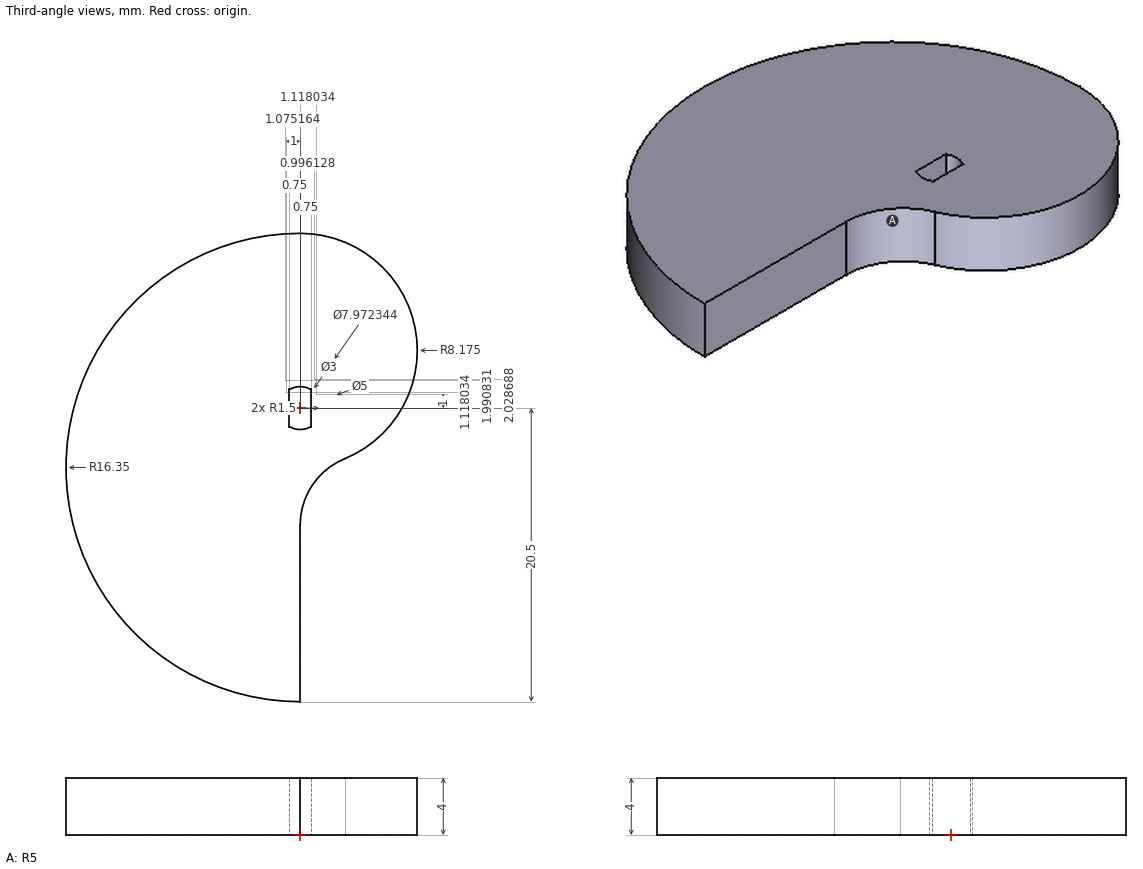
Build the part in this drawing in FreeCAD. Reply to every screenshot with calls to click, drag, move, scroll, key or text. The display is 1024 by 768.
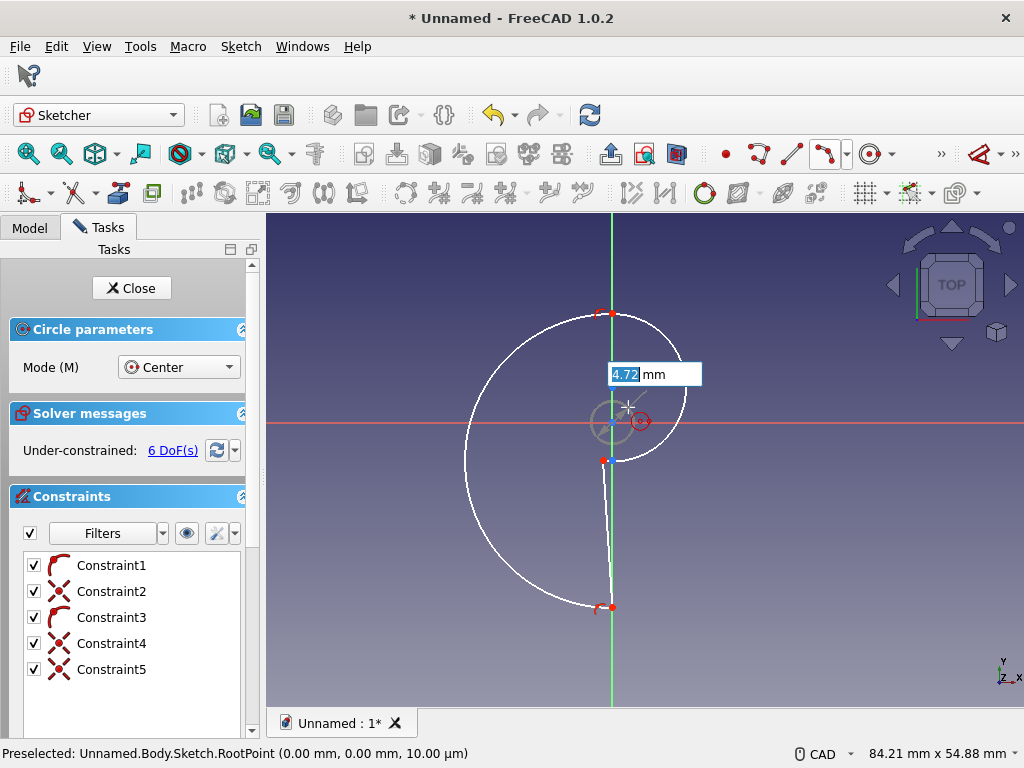
text(5)
key(Return)
key(Escape)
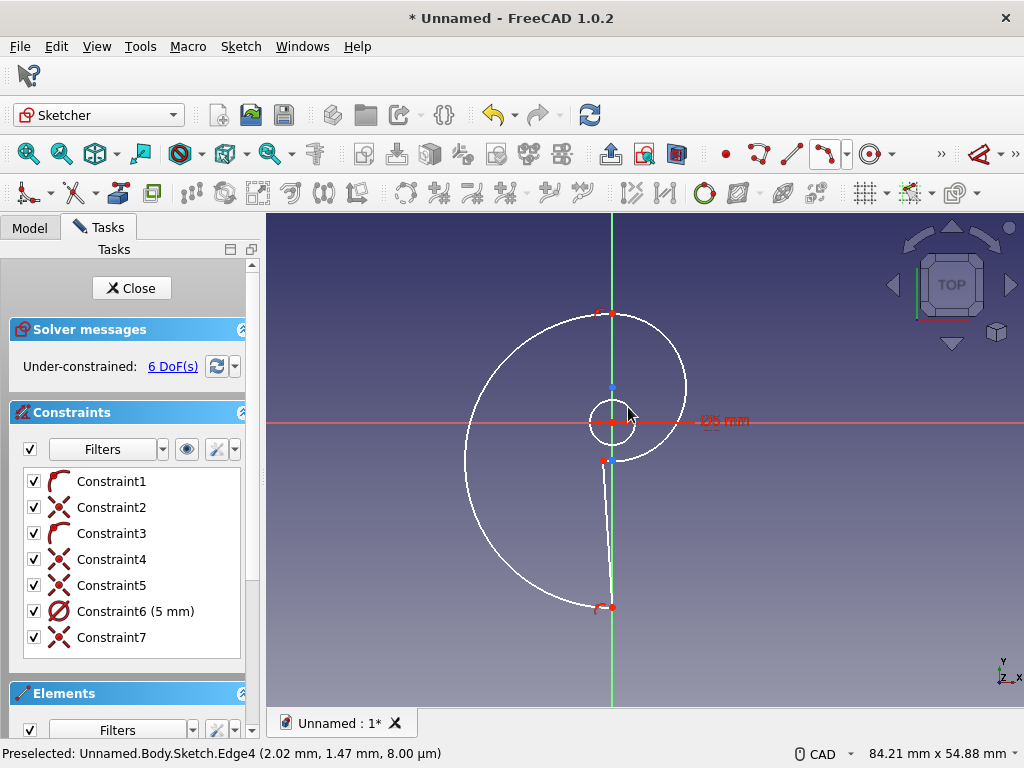
click(668, 436)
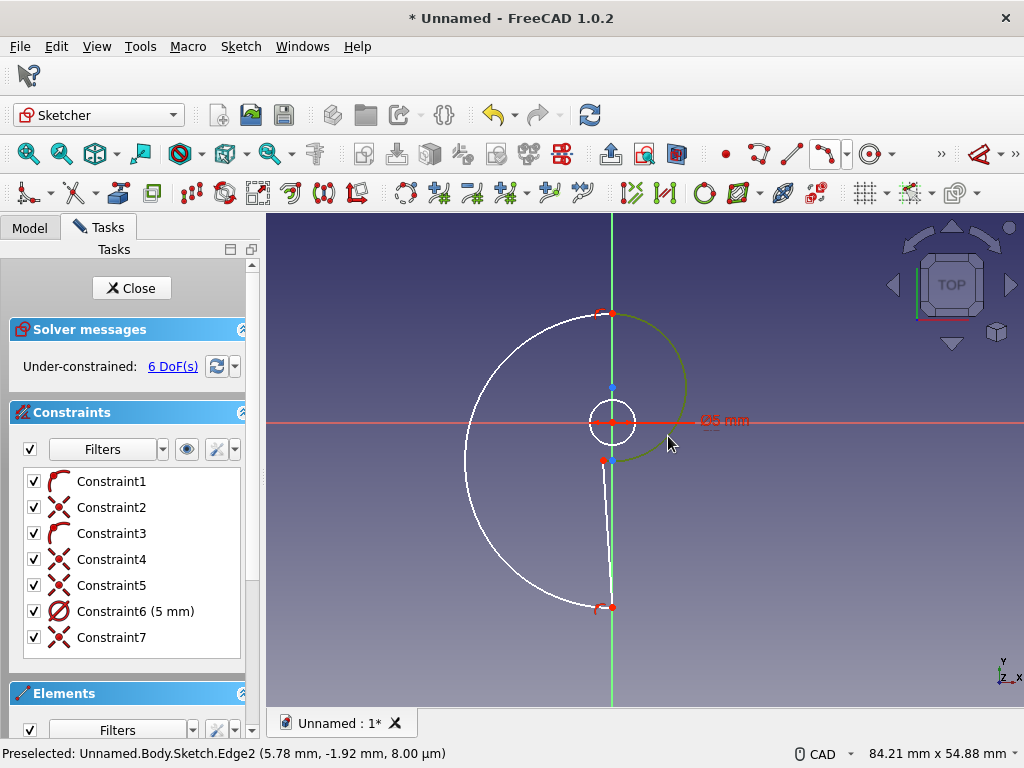
click(493, 374)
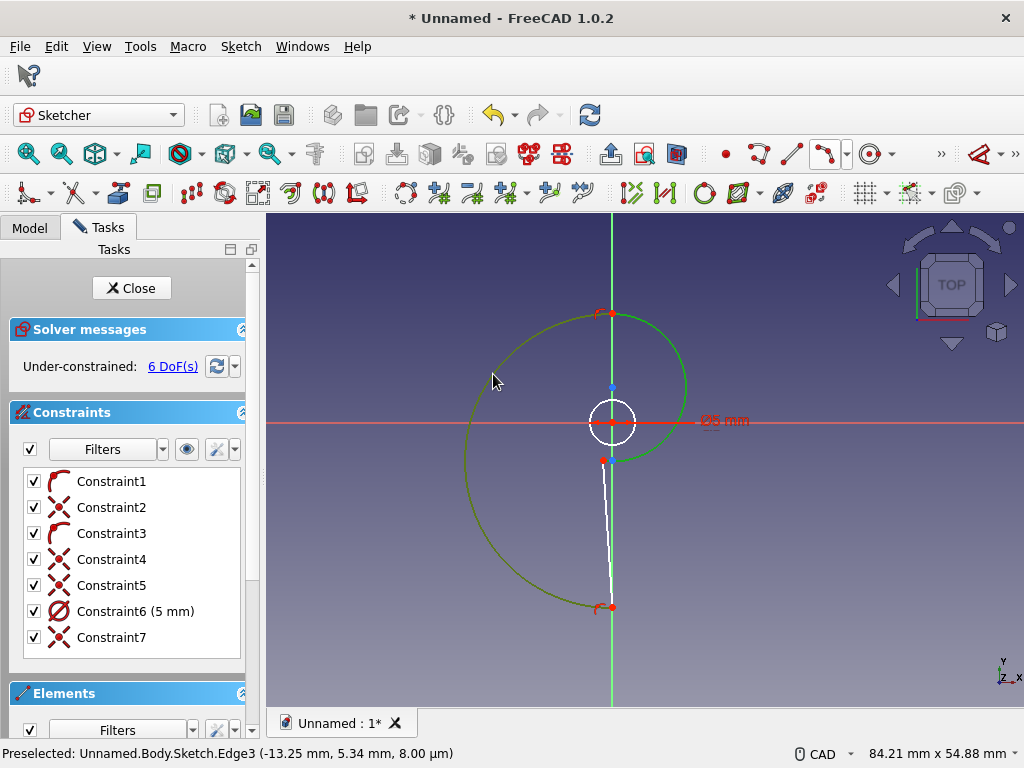
key(t)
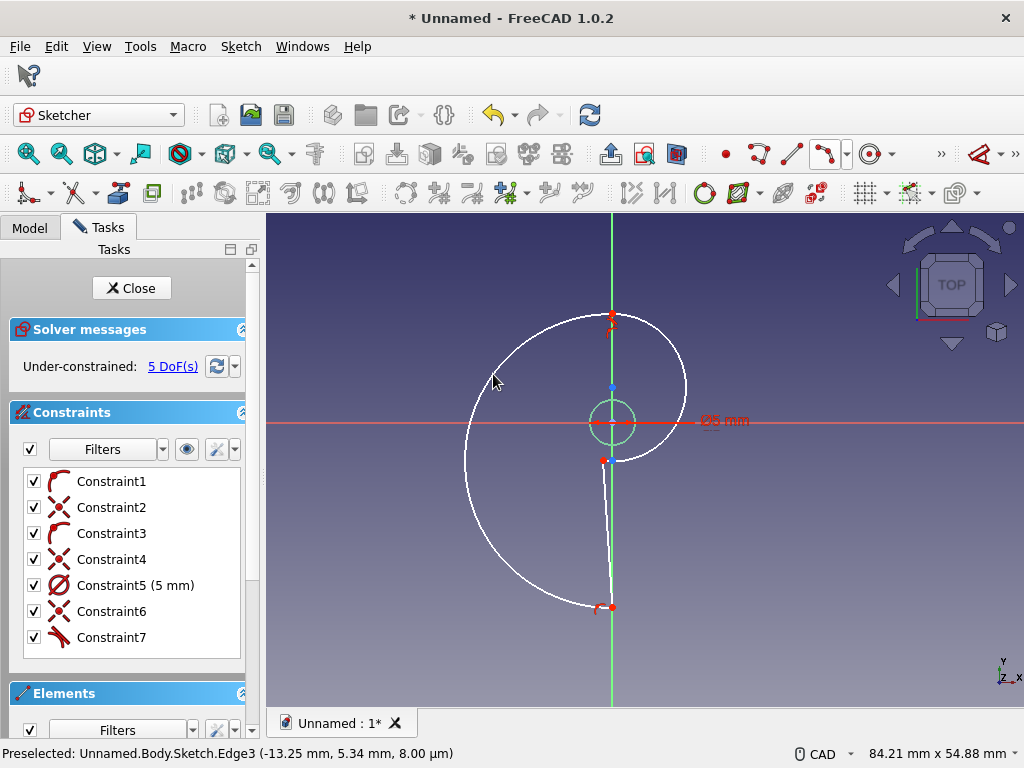
click(610, 564)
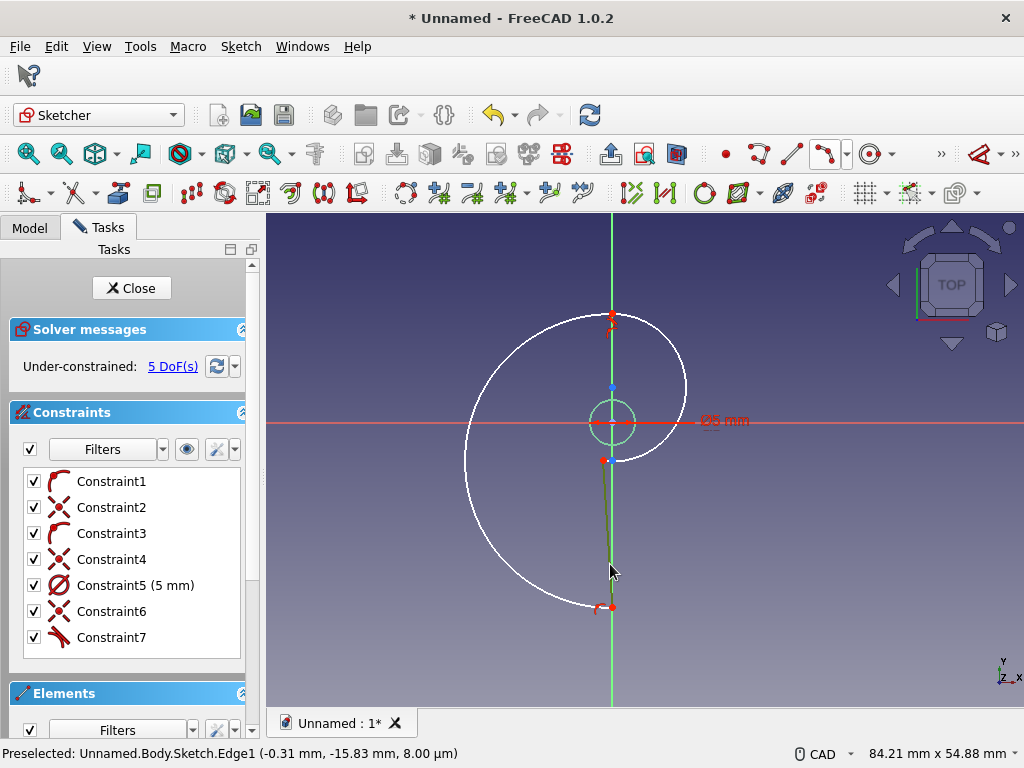
key(v)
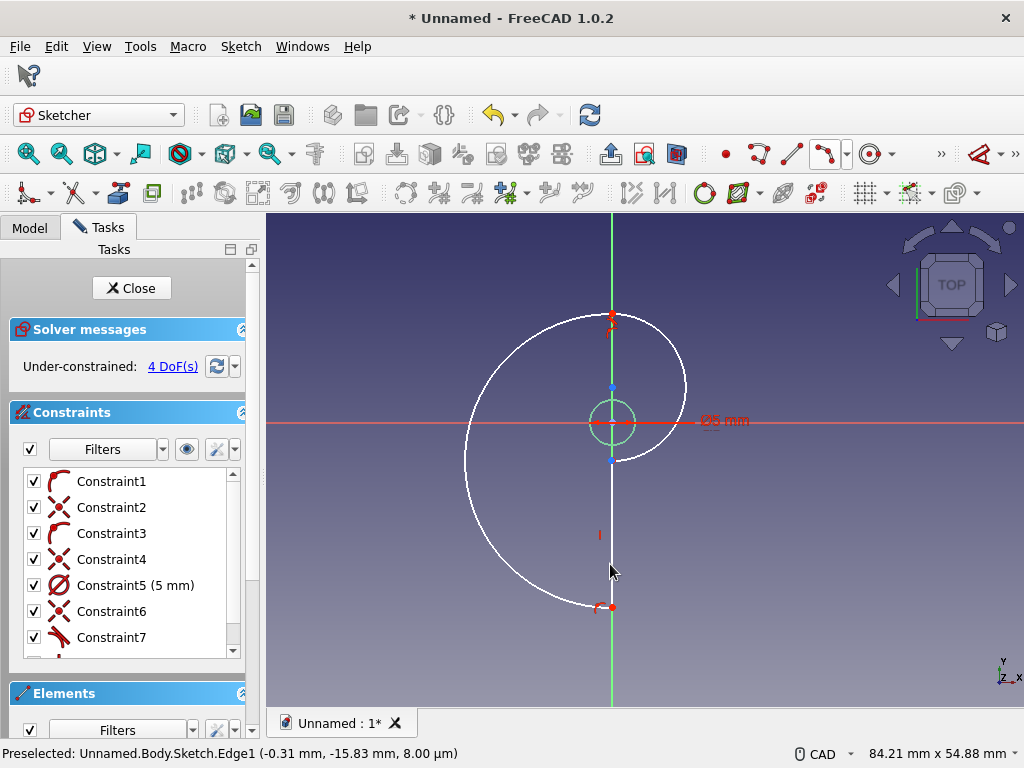
click(612, 387)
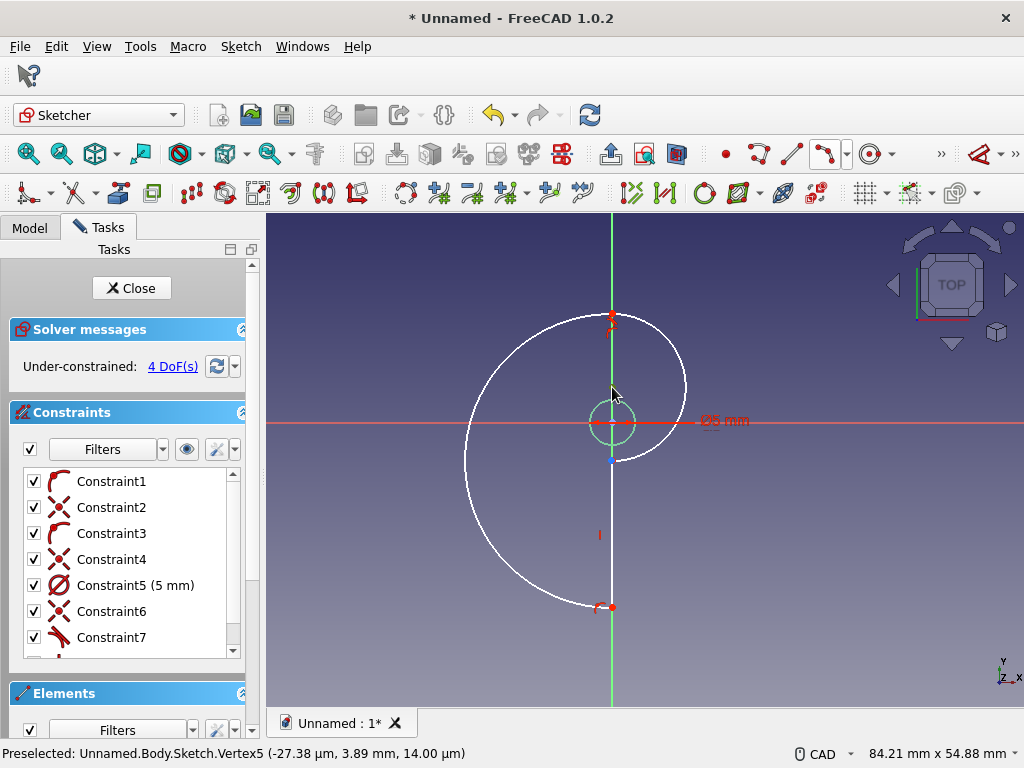
click(612, 648)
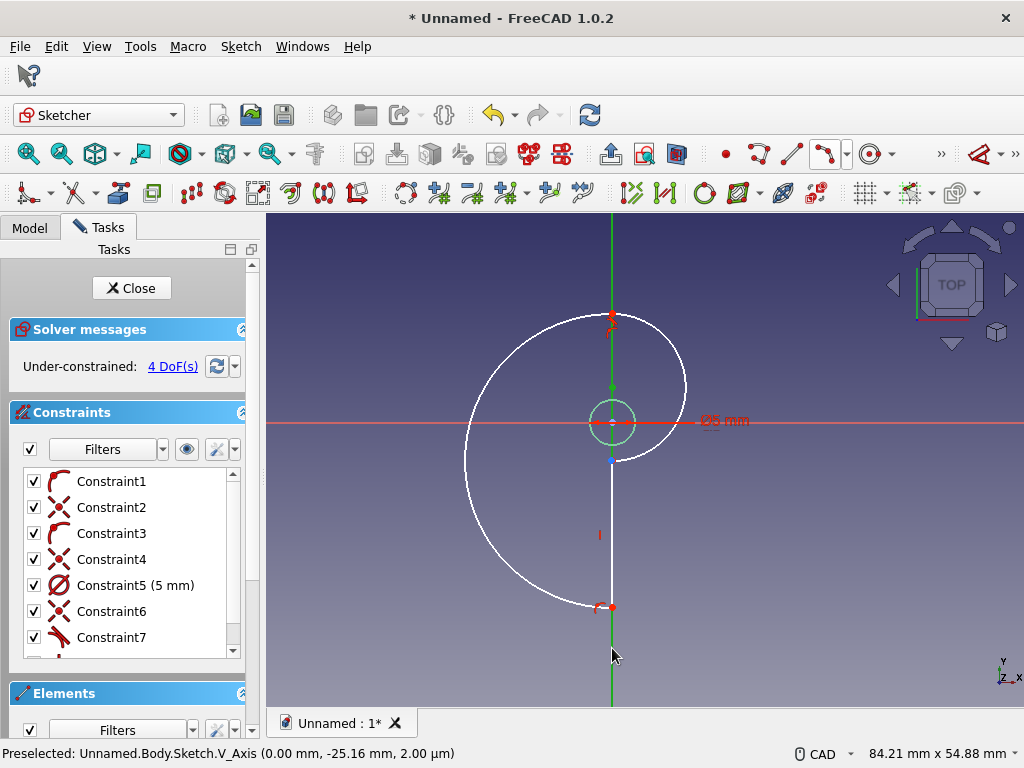
key(c)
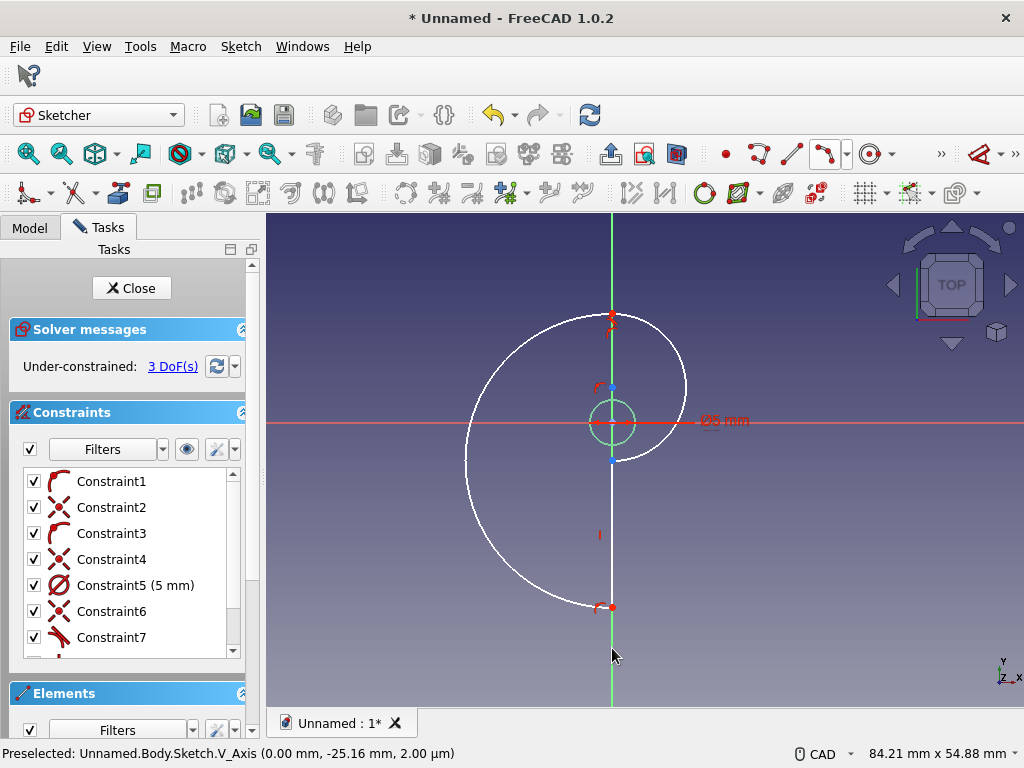
click(978, 154)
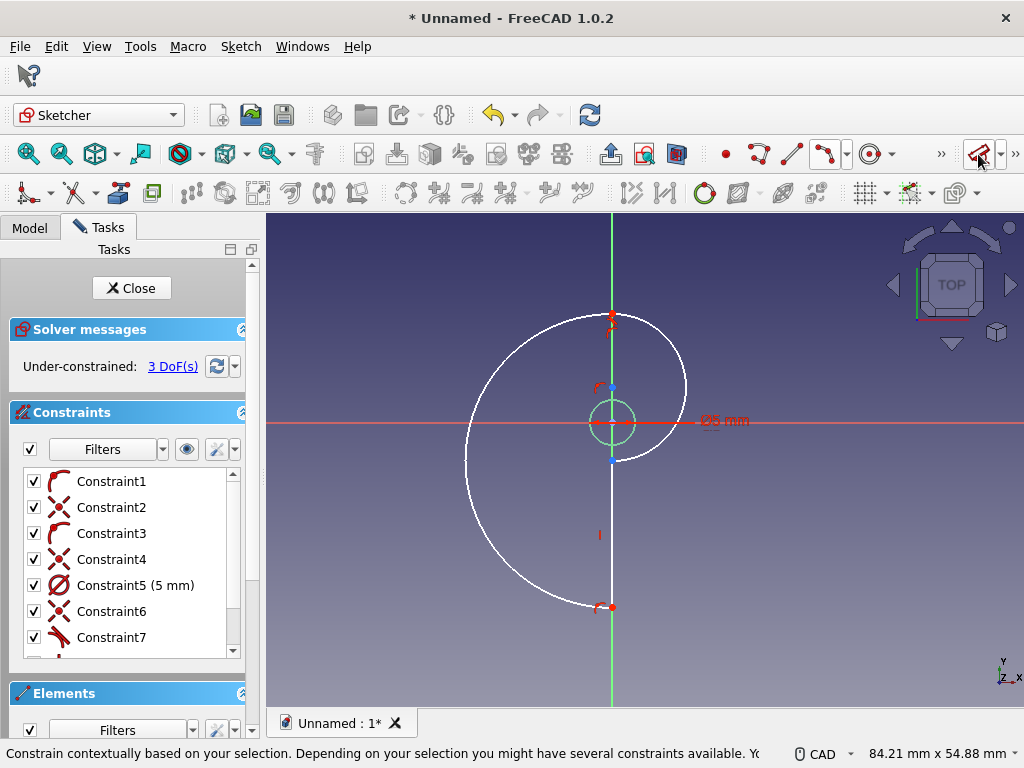
click(672, 344)
click(698, 325)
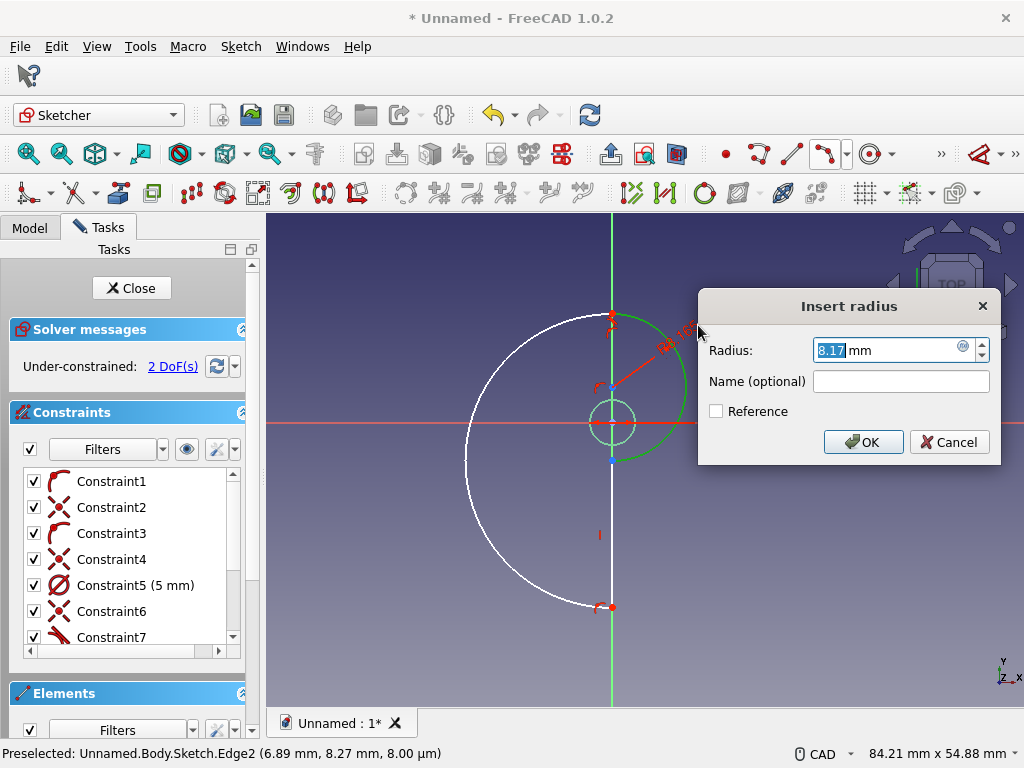
text(8.175)
key(Return)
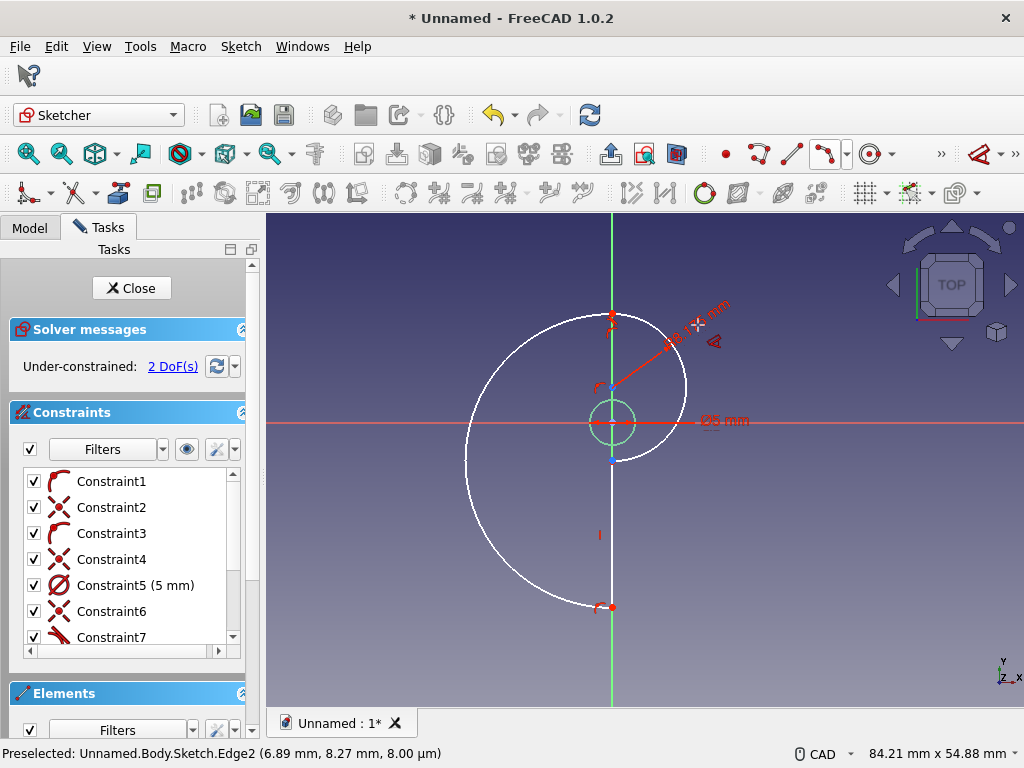
click(494, 375)
click(468, 356)